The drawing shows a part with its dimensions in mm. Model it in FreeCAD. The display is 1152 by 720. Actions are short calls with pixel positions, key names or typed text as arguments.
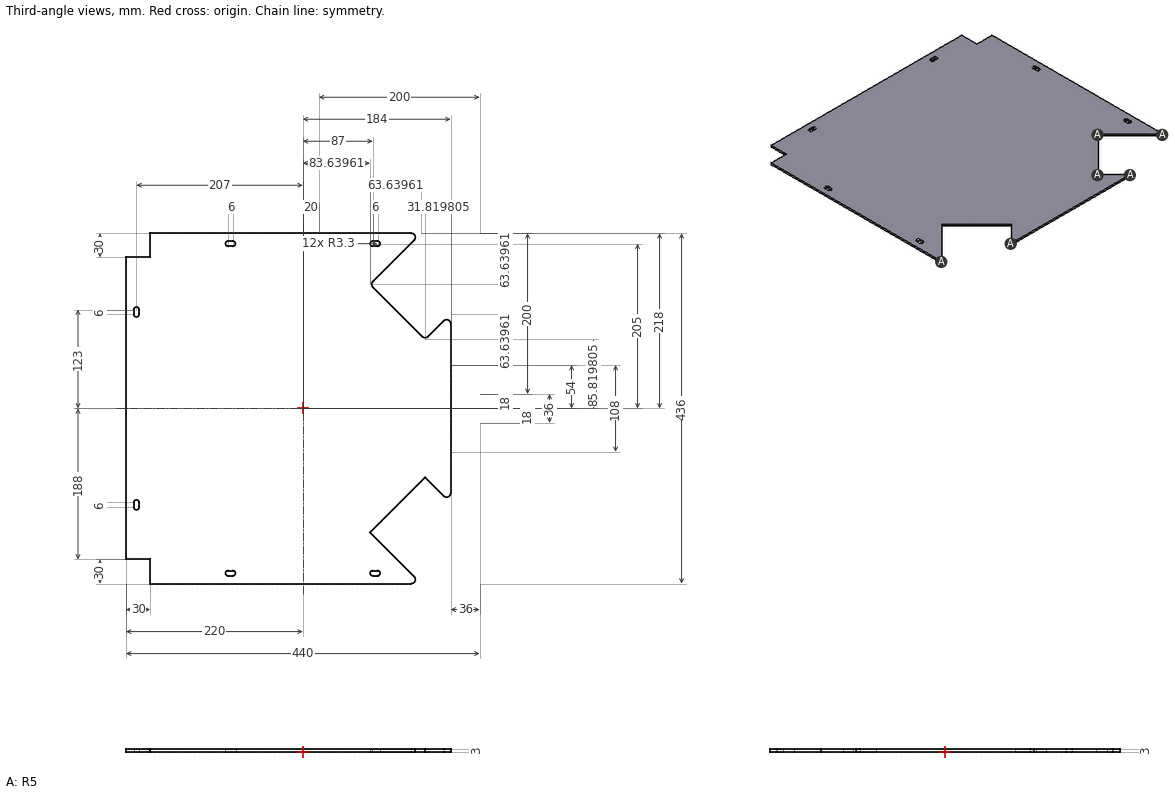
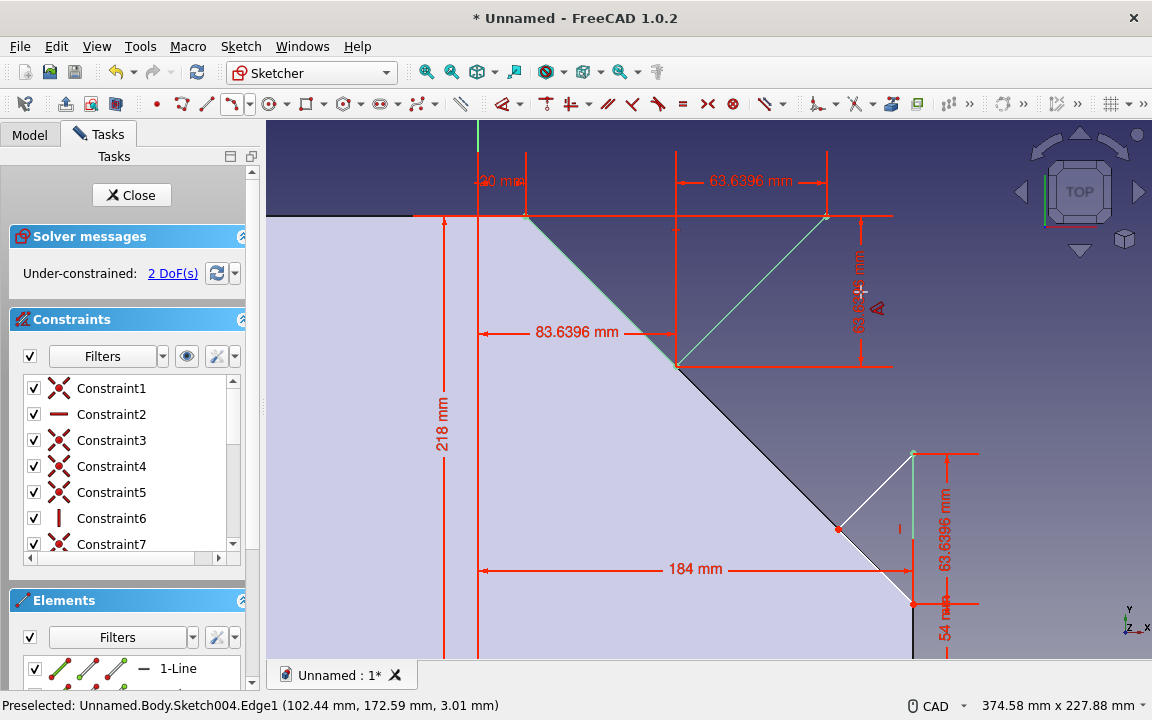
click(838, 530)
click(444, 580)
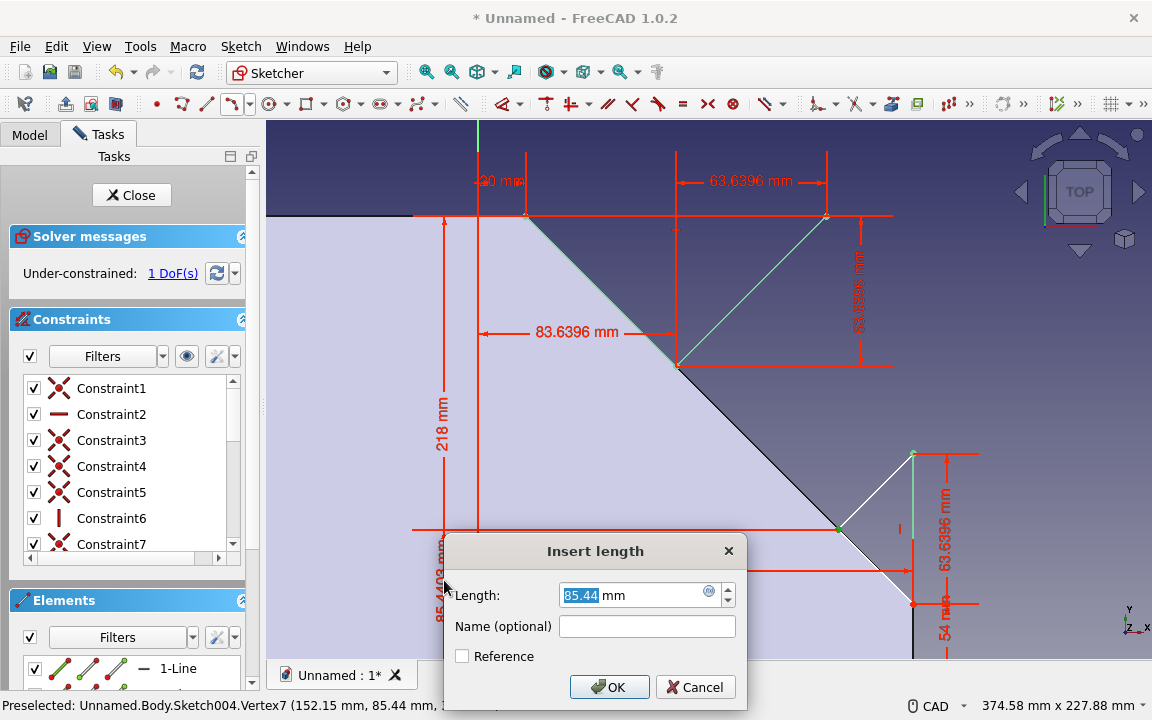
text(85.819805)
key(Return)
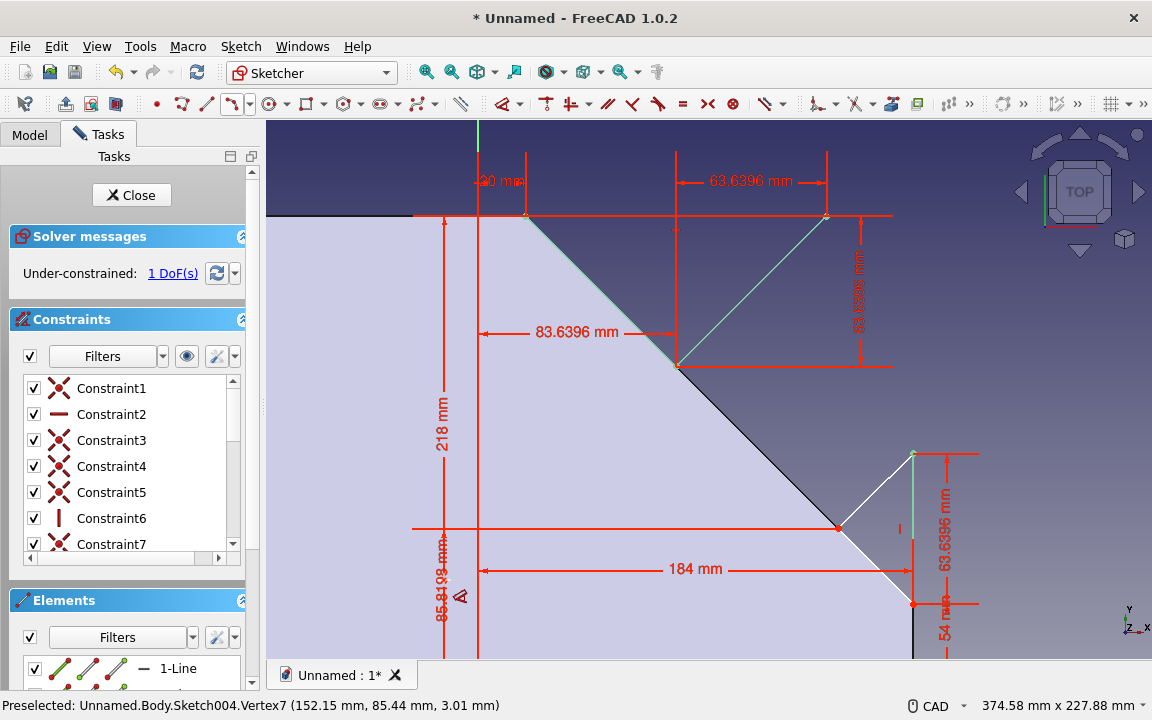
click(861, 551)
click(893, 495)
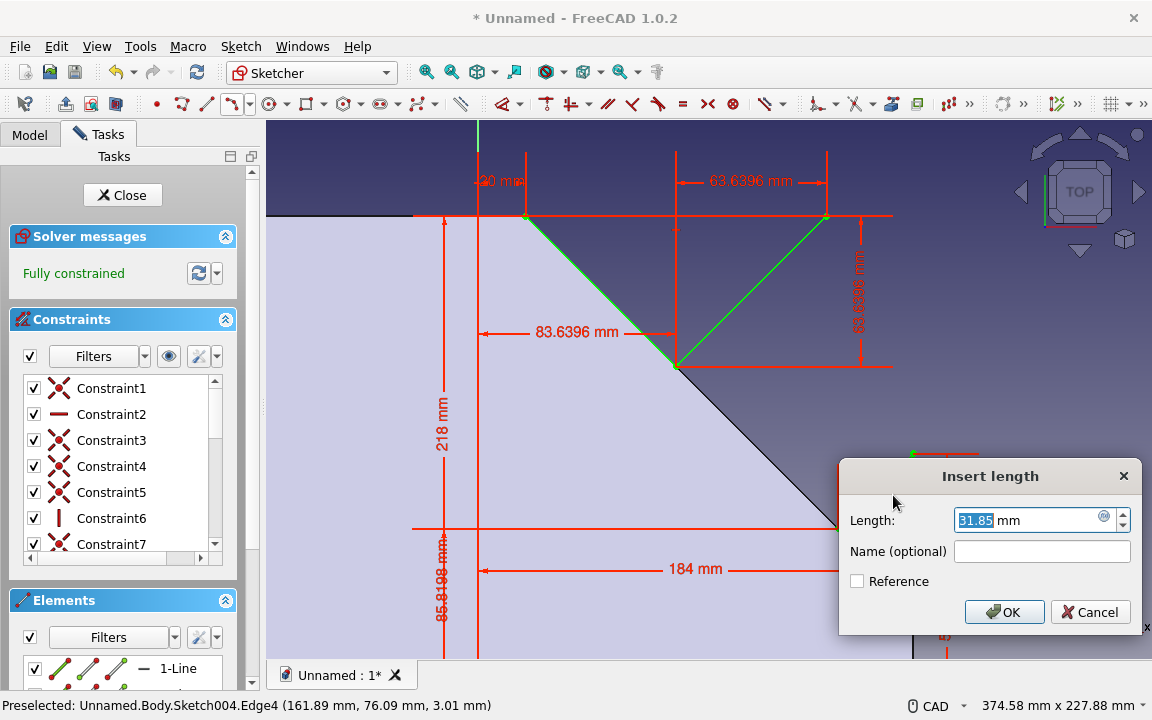
text(31.819805)
key(Return)
key(Escape)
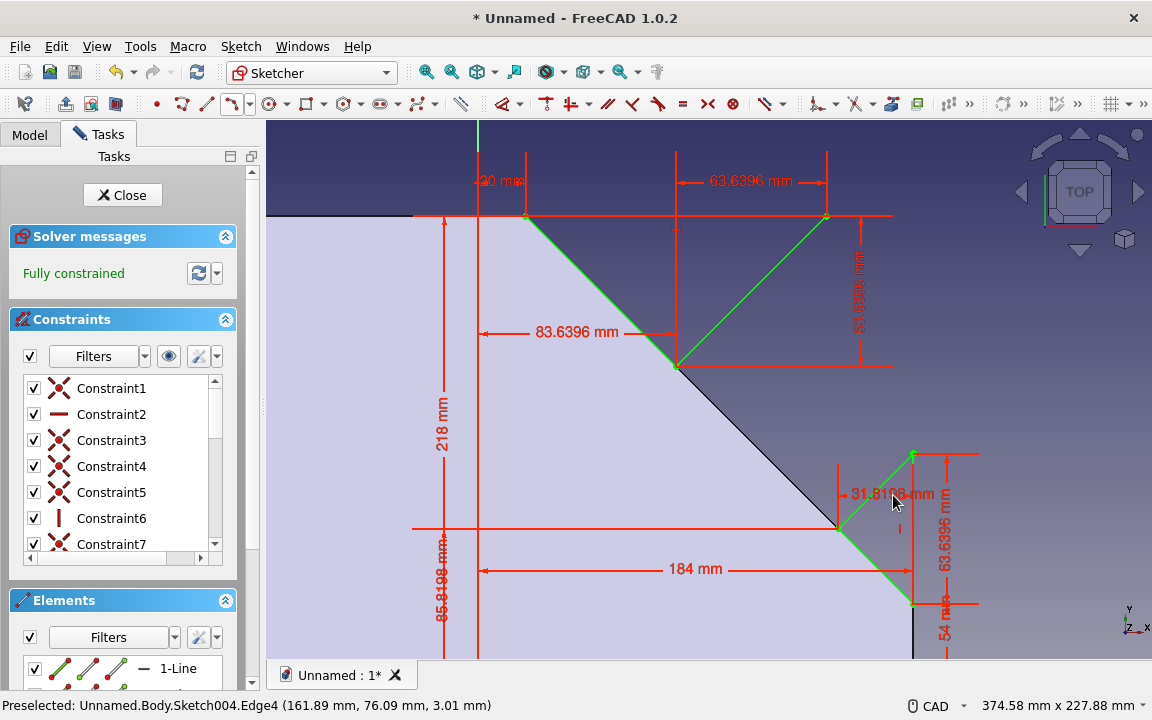
click(123, 195)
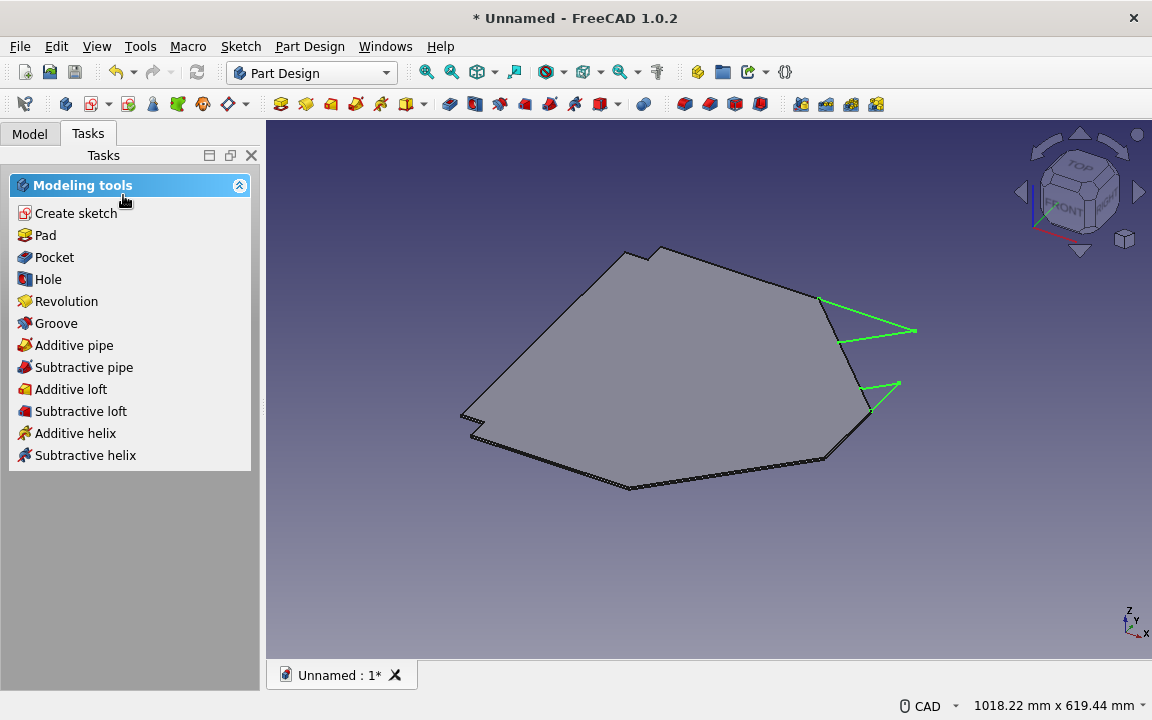
click(281, 104)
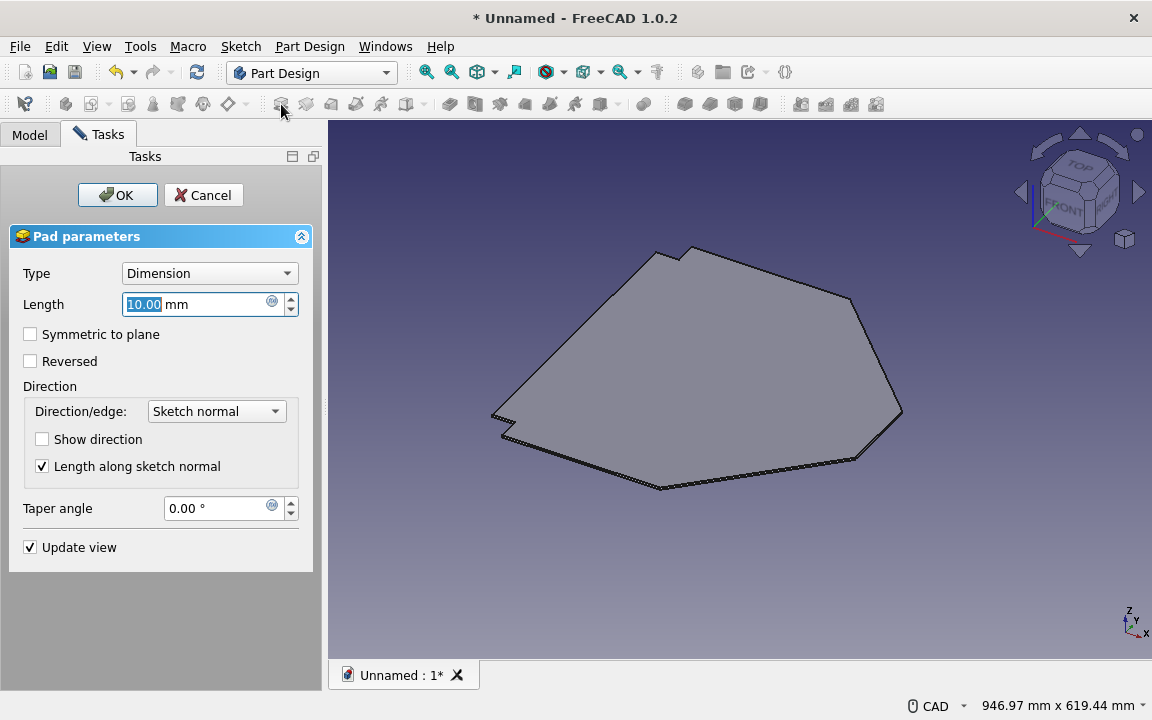
text(3)
key(Tab)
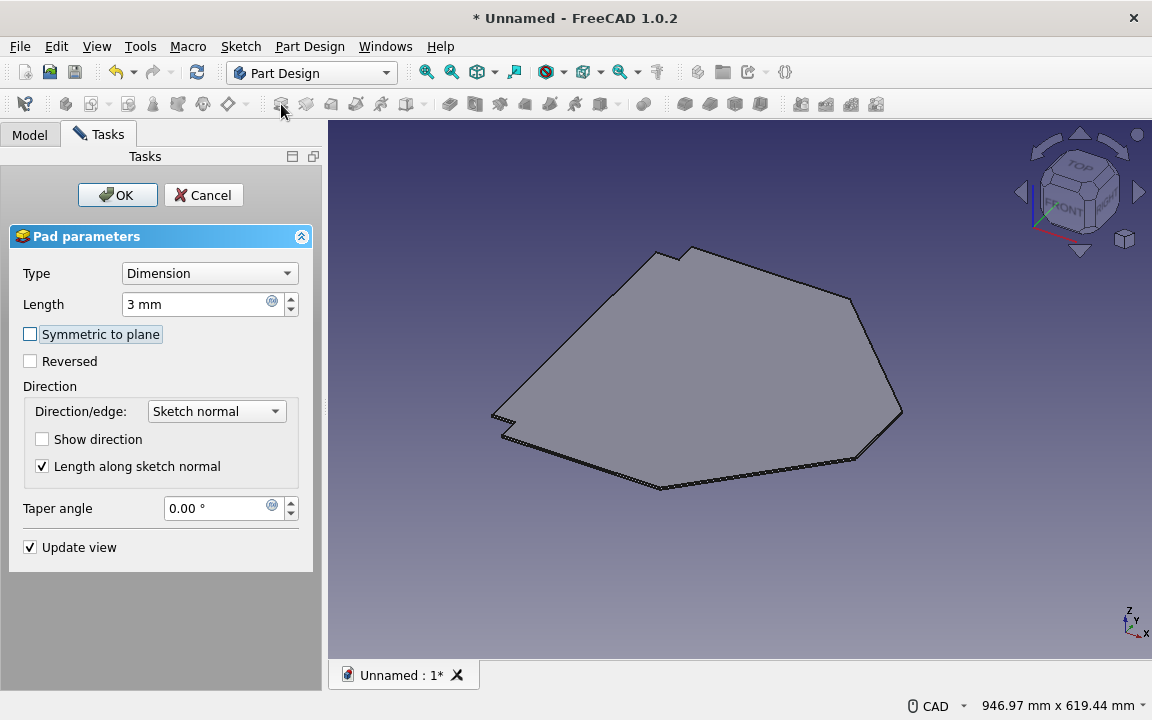
click(31, 361)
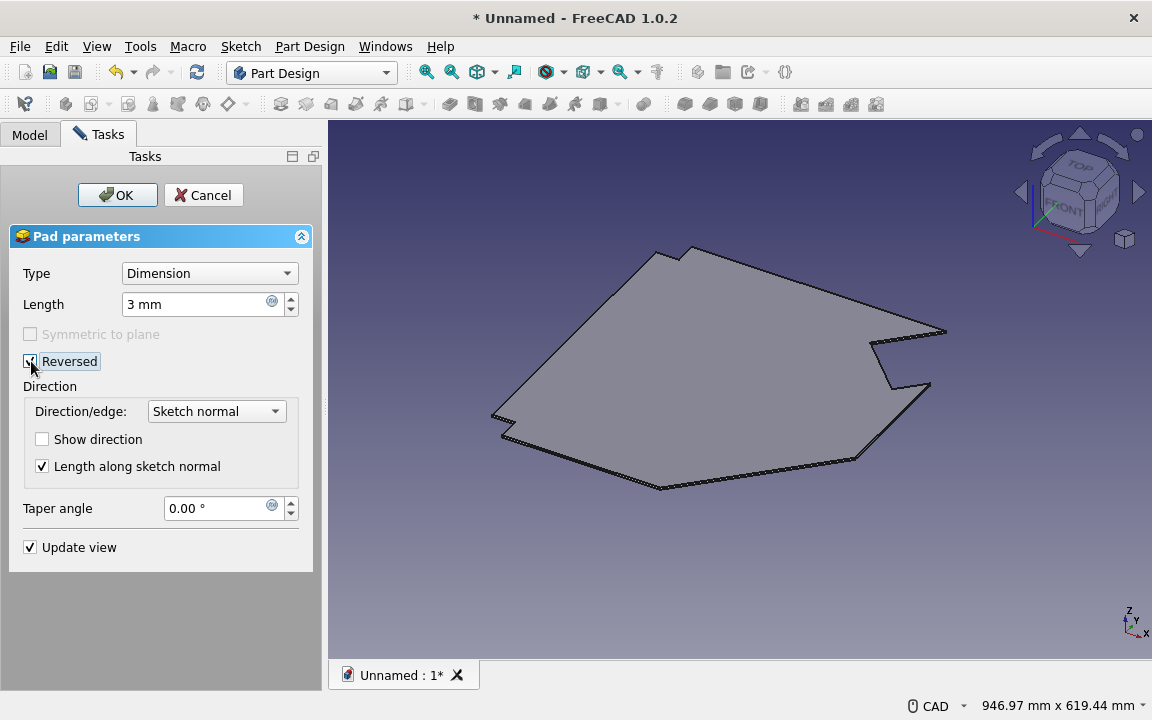
click(118, 195)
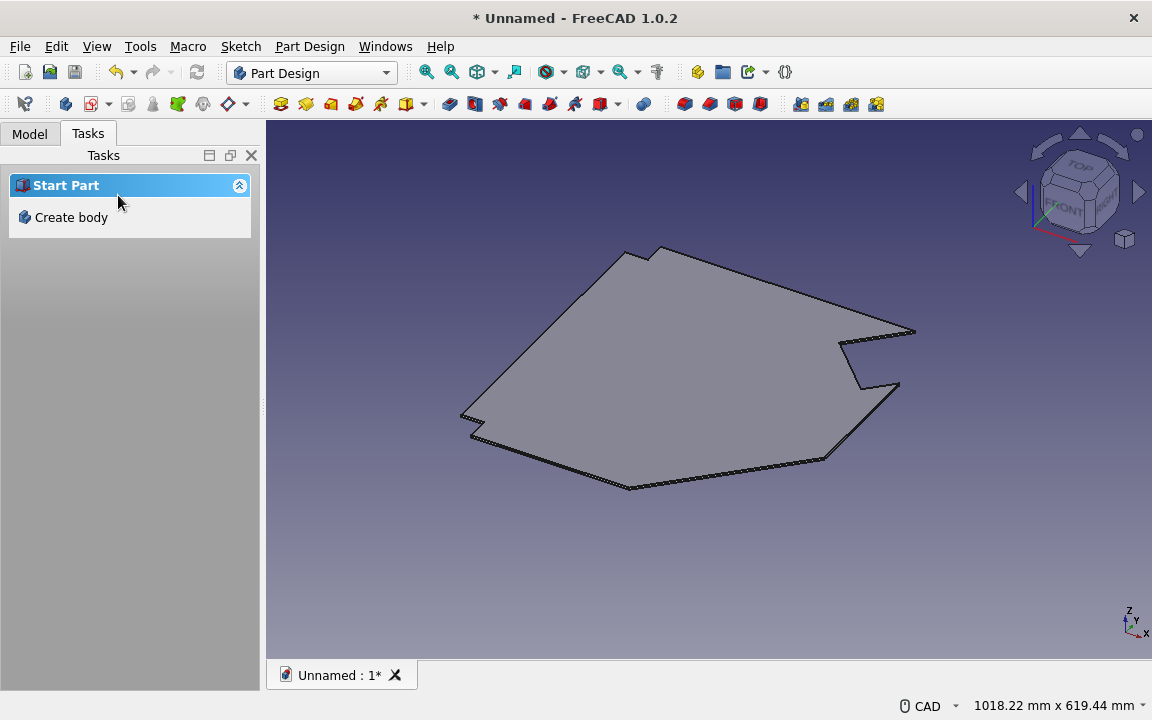
click(30, 134)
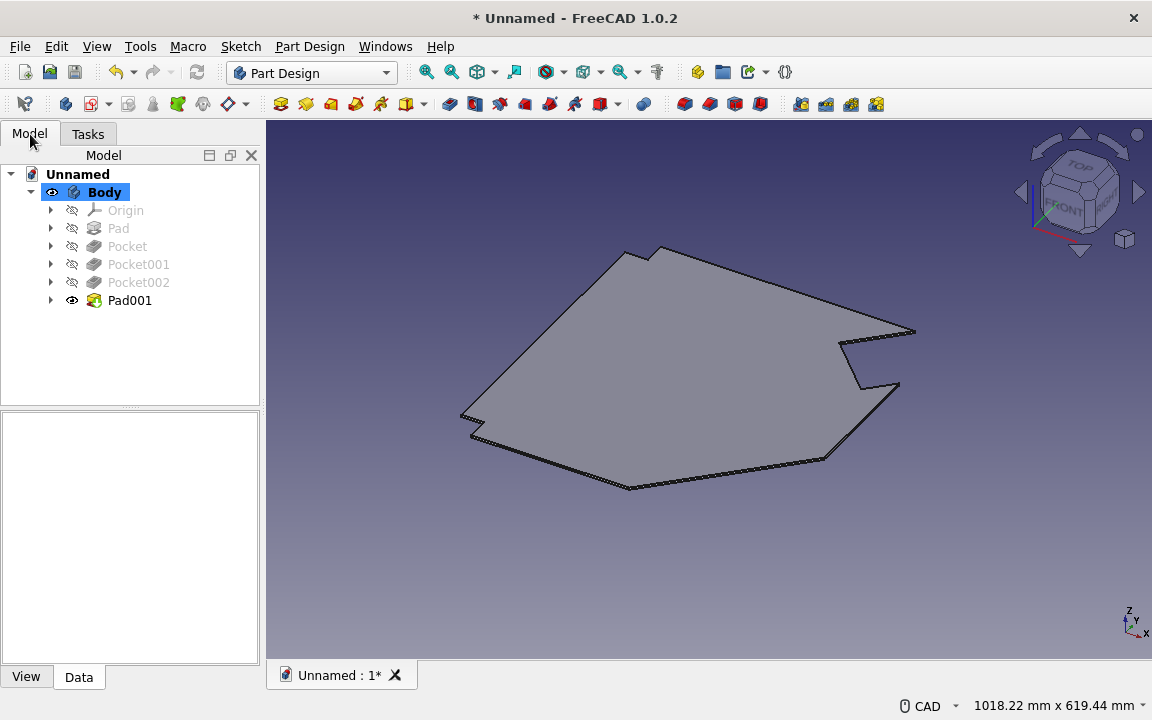
click(117, 300)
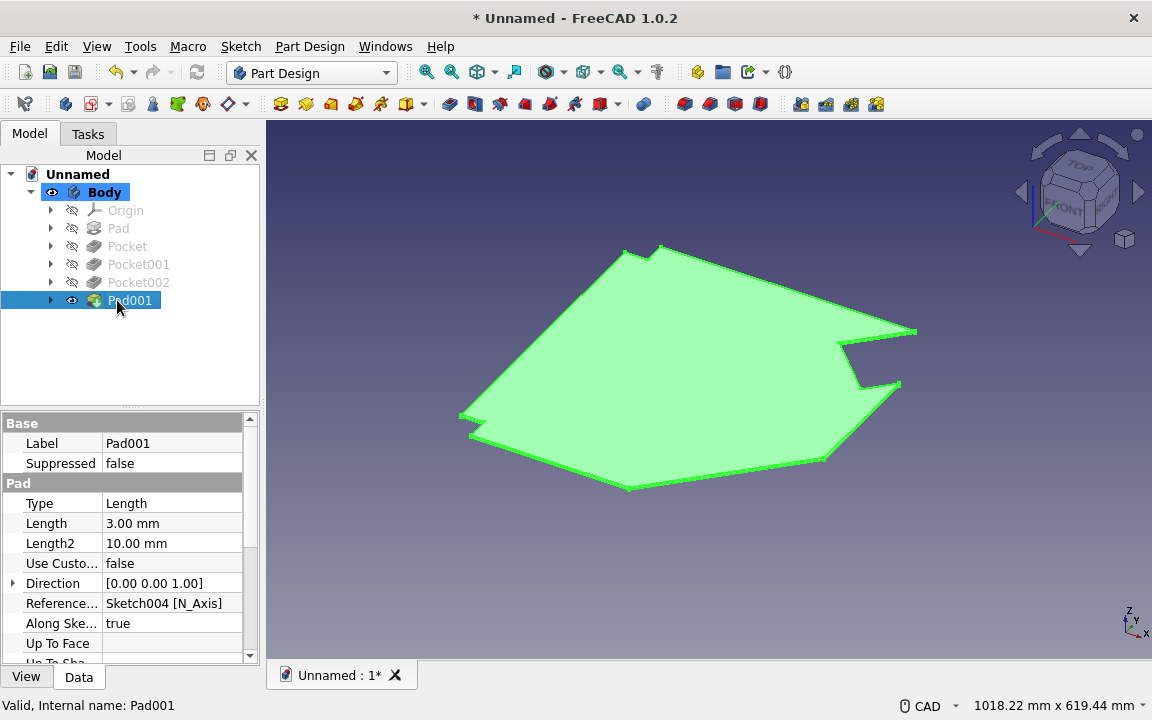
click(801, 104)